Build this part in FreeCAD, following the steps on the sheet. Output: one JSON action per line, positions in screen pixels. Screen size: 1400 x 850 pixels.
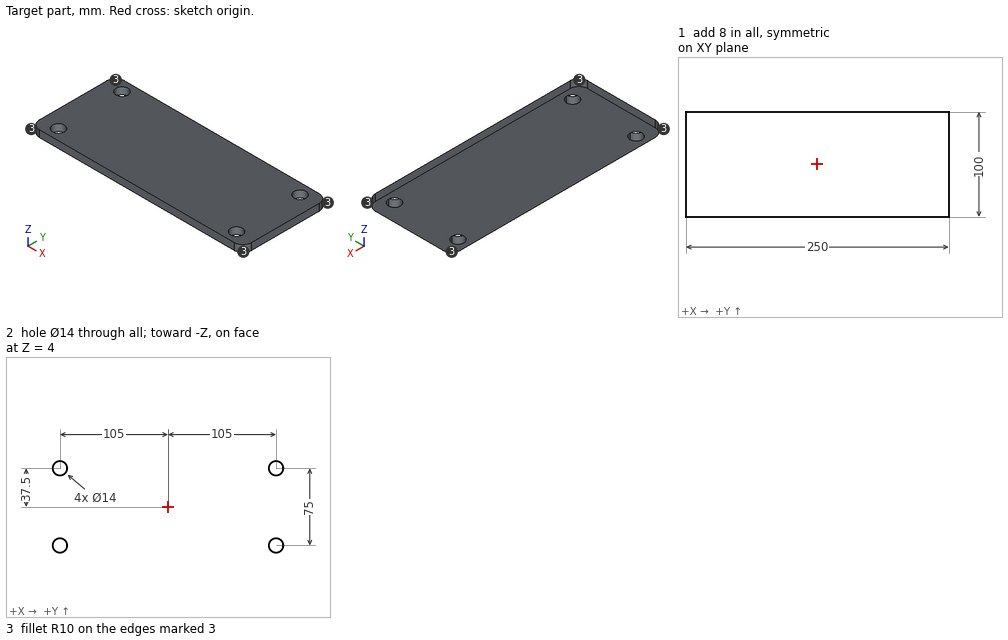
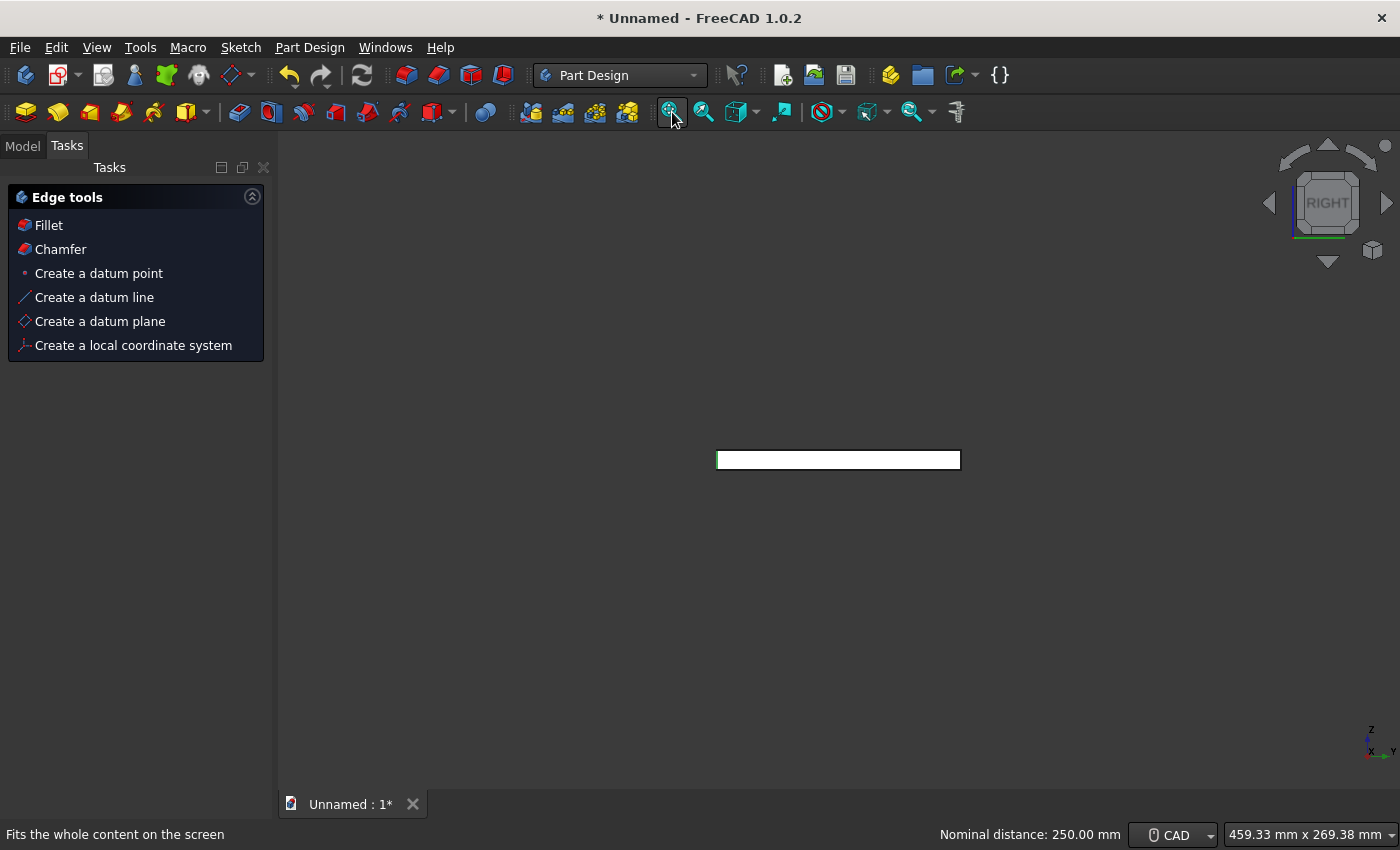
{"action": "left_click", "coordinate": [672, 112]}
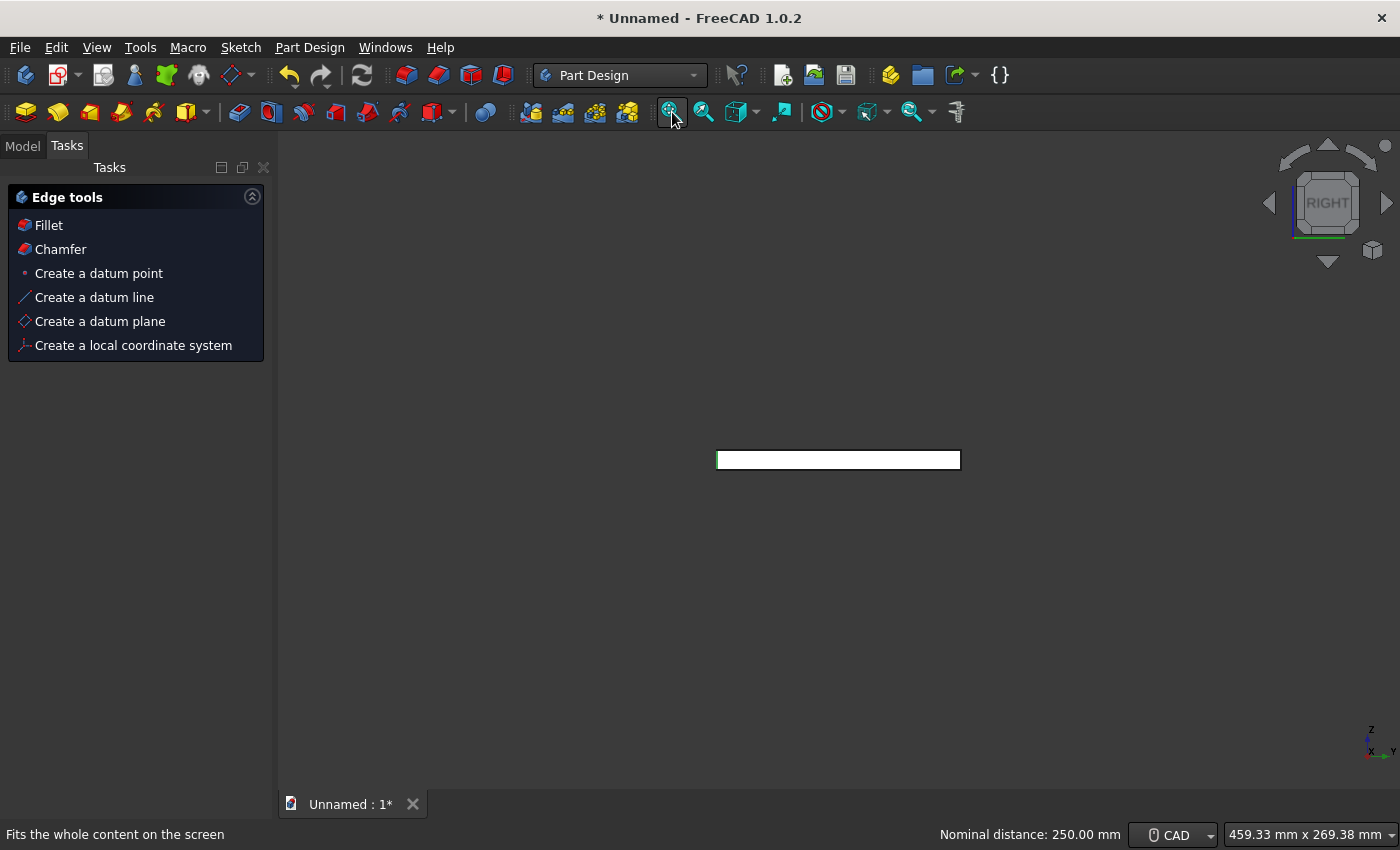
{"action": "left_click", "coordinate": [961, 459], "text": "ctrl"}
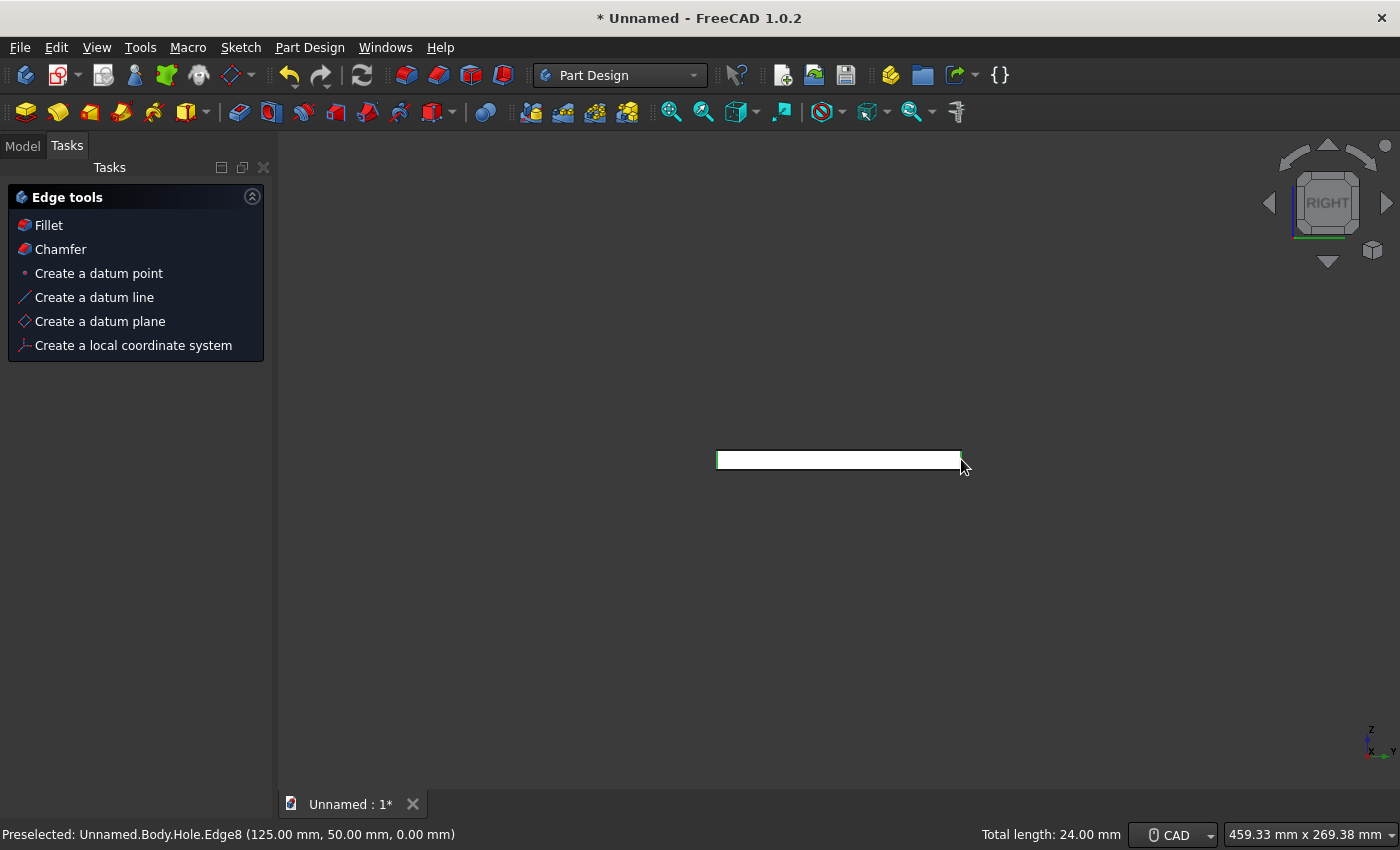
{"action": "scroll", "coordinate": [961, 459], "scroll_direction": "up", "scroll_amount": 4}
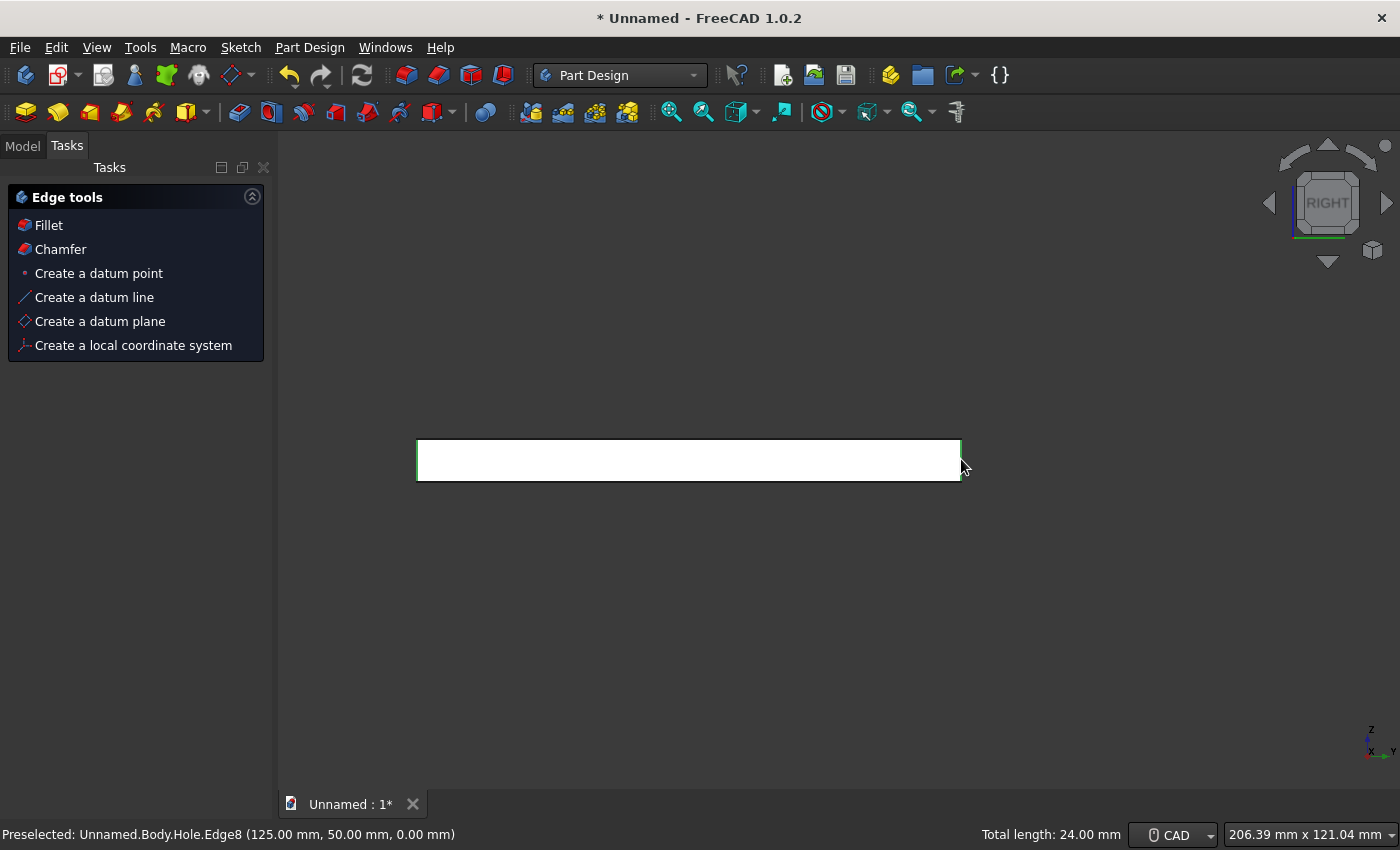
{"action": "left_click", "coordinate": [672, 112]}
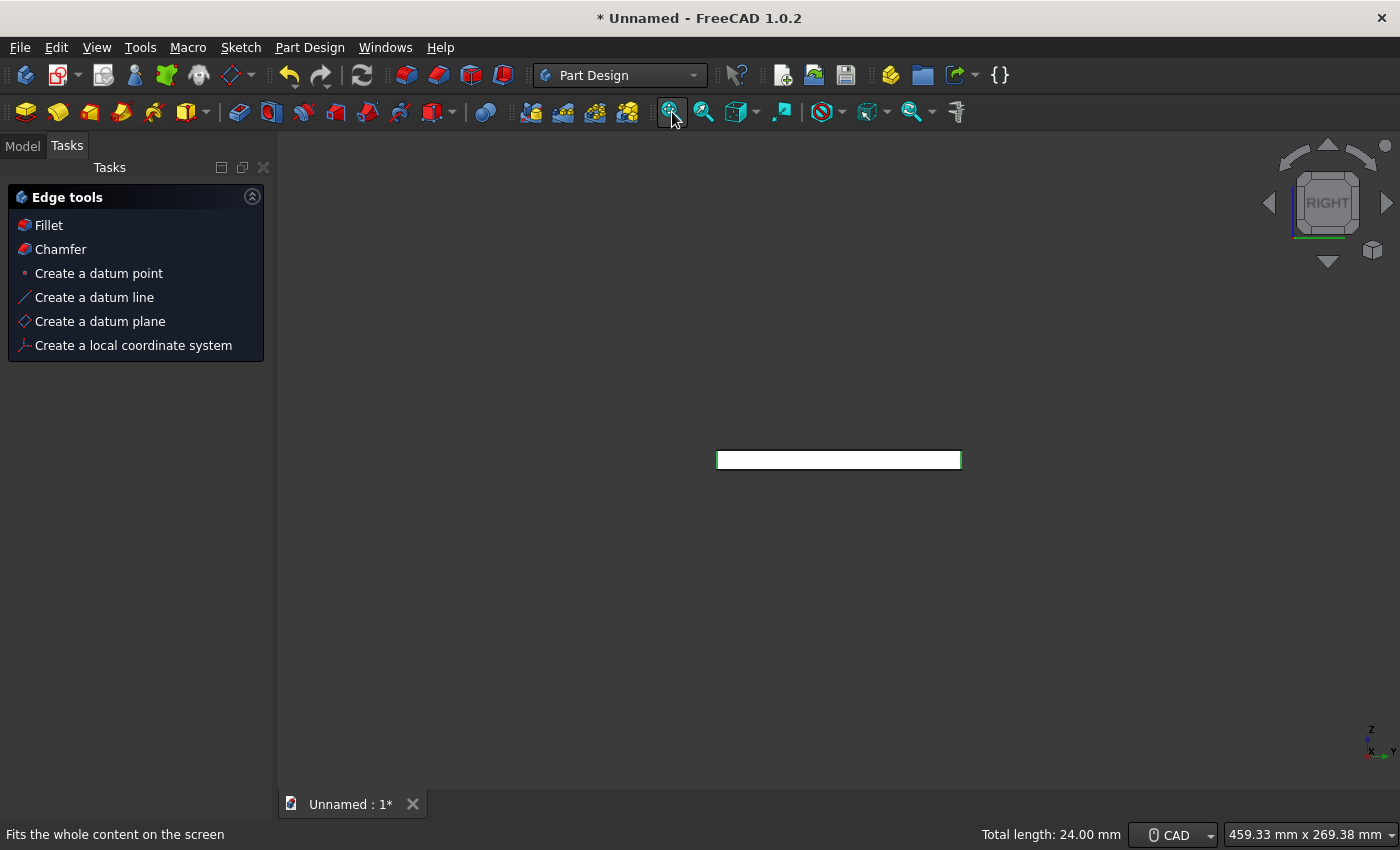
{"action": "key", "text": "5"}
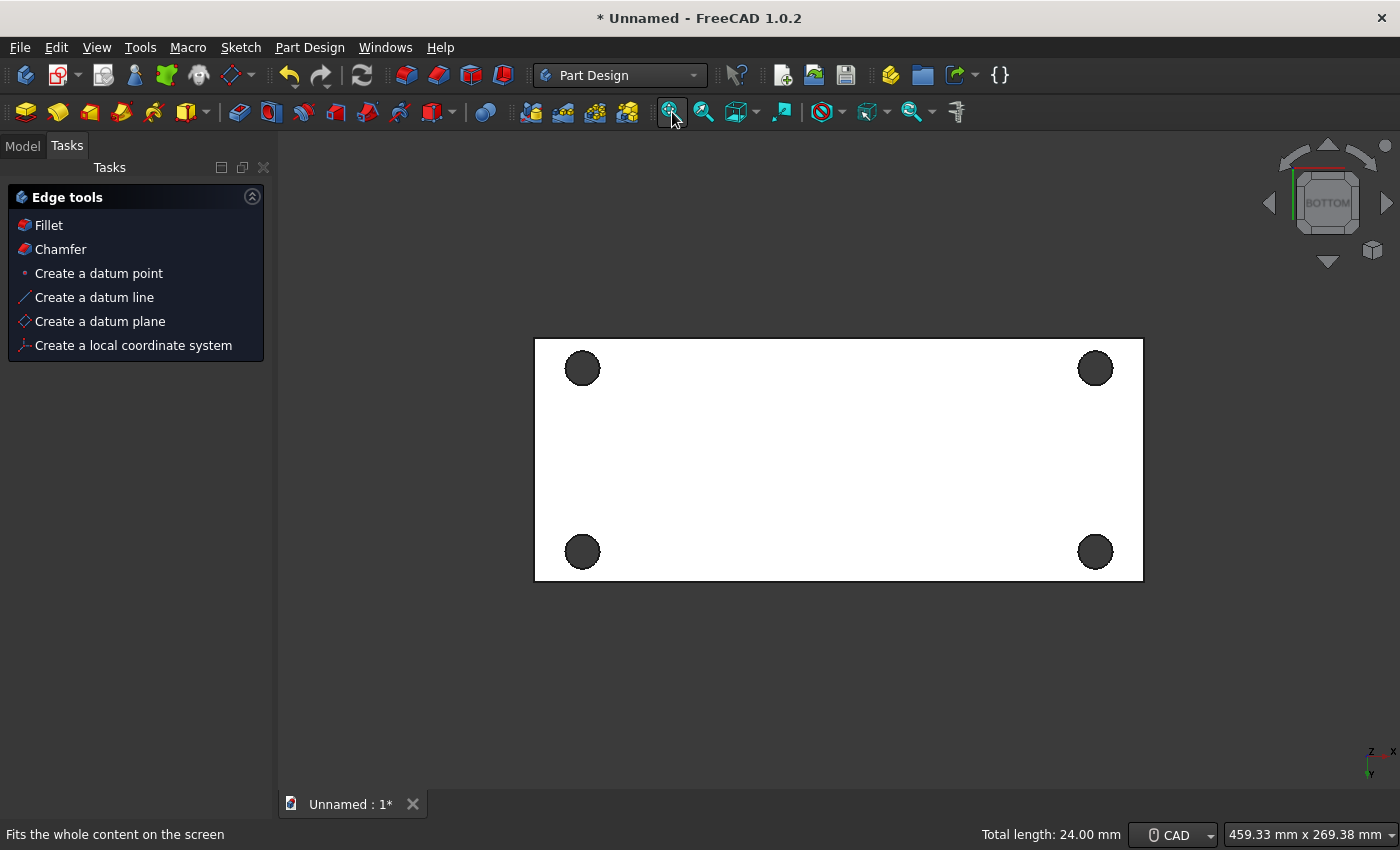
{"action": "scroll", "coordinate": [534, 581], "scroll_direction": "up", "scroll_amount": 4}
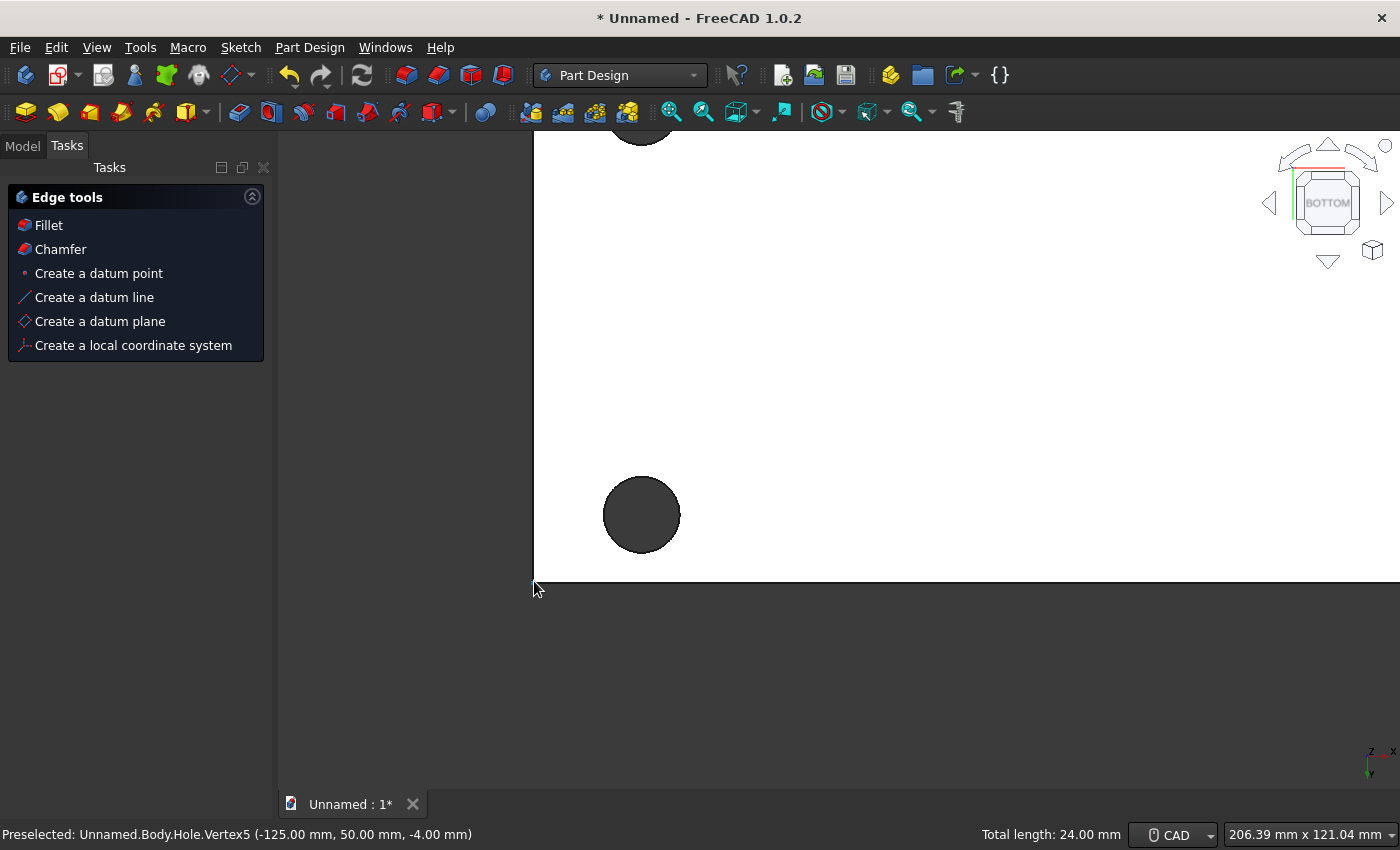
{"action": "left_click", "coordinate": [672, 112]}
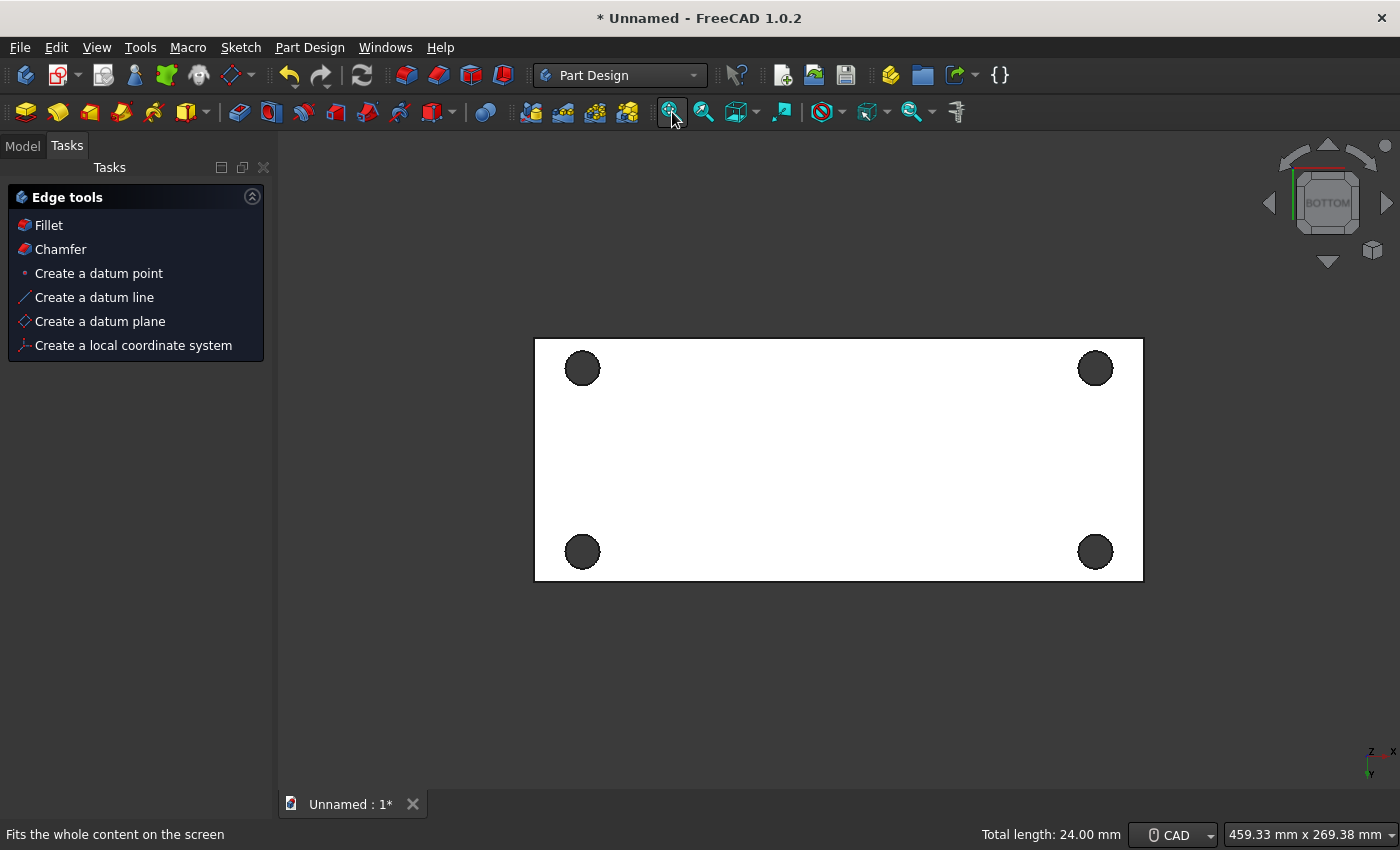
{"action": "key", "text": "4"}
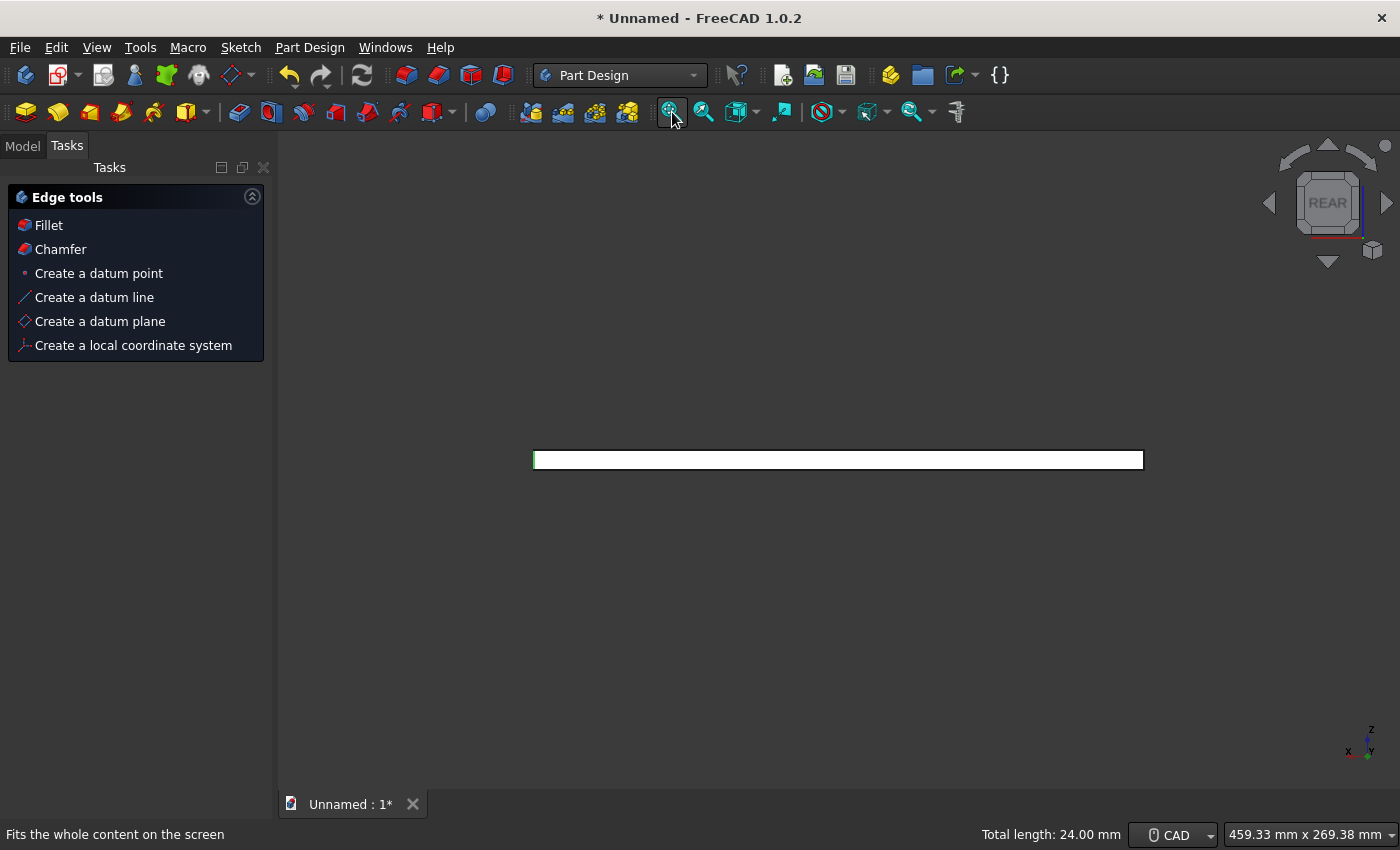
{"action": "left_click", "coordinate": [1144, 459], "text": "ctrl"}